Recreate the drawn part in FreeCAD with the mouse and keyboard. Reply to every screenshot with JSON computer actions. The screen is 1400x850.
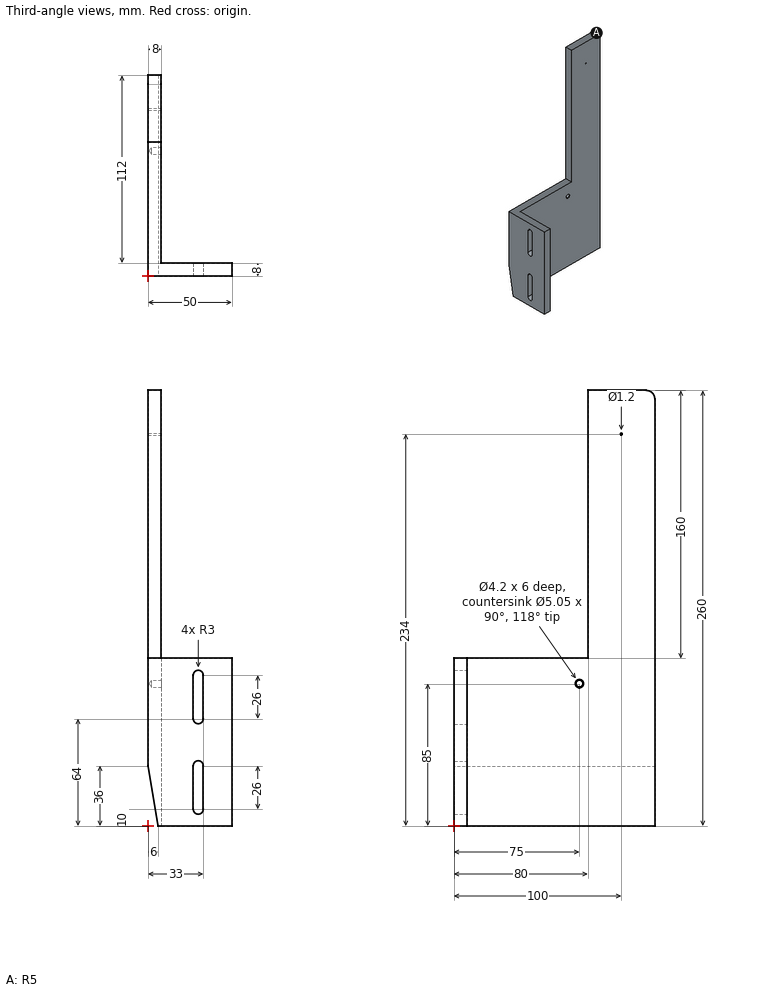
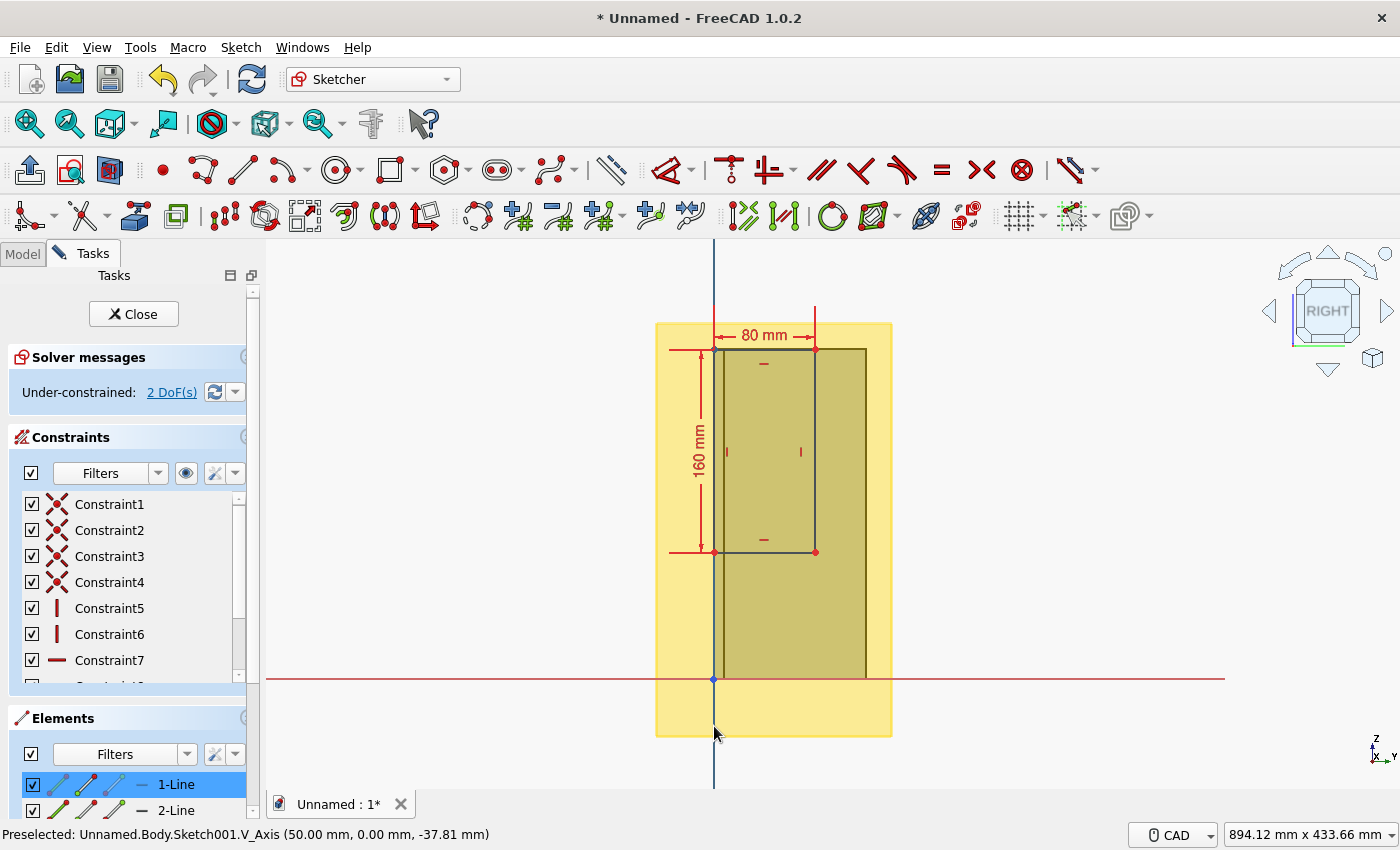
{"action": "left_click", "coordinate": [730, 170]}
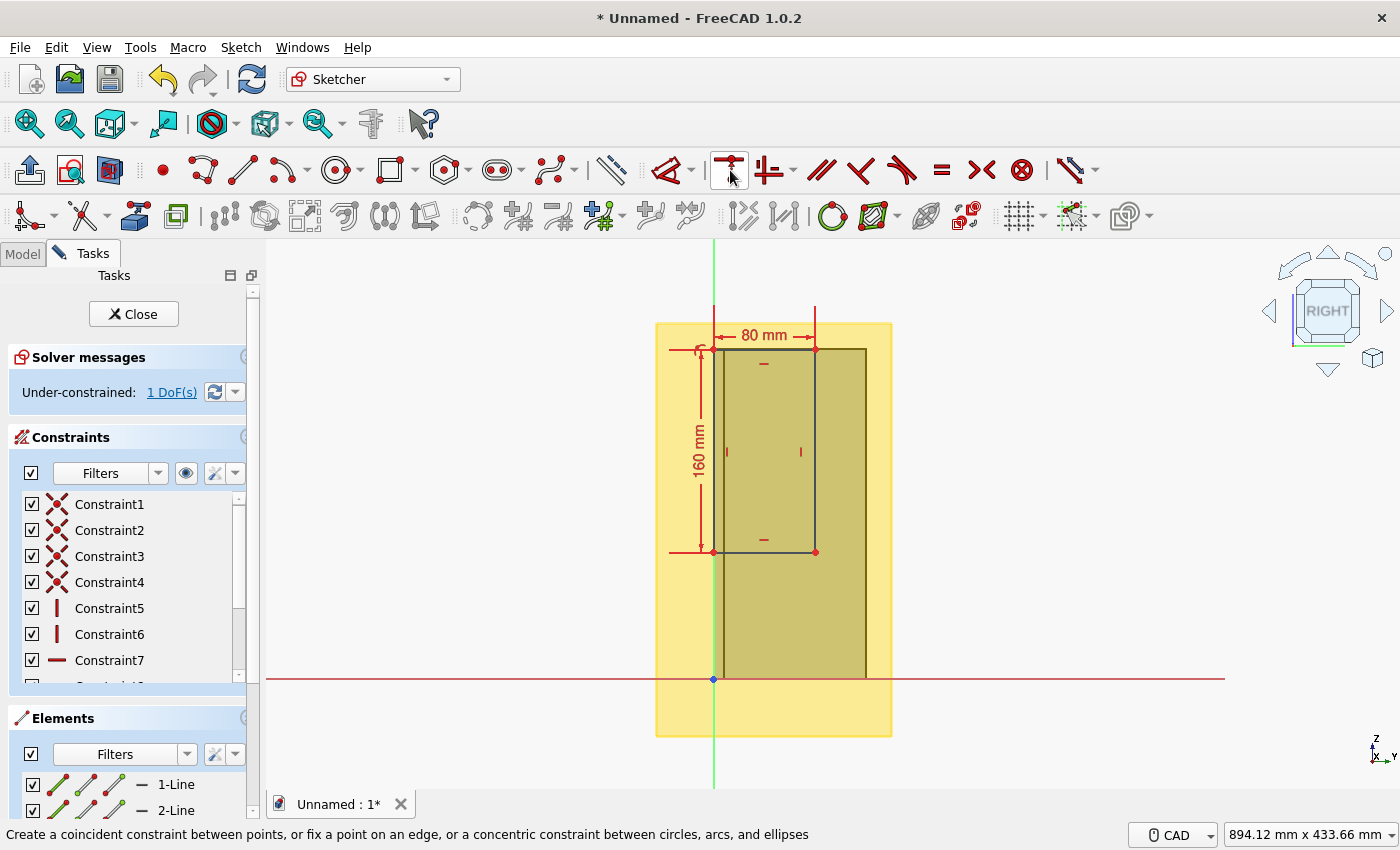
{"action": "left_click", "coordinate": [666, 170]}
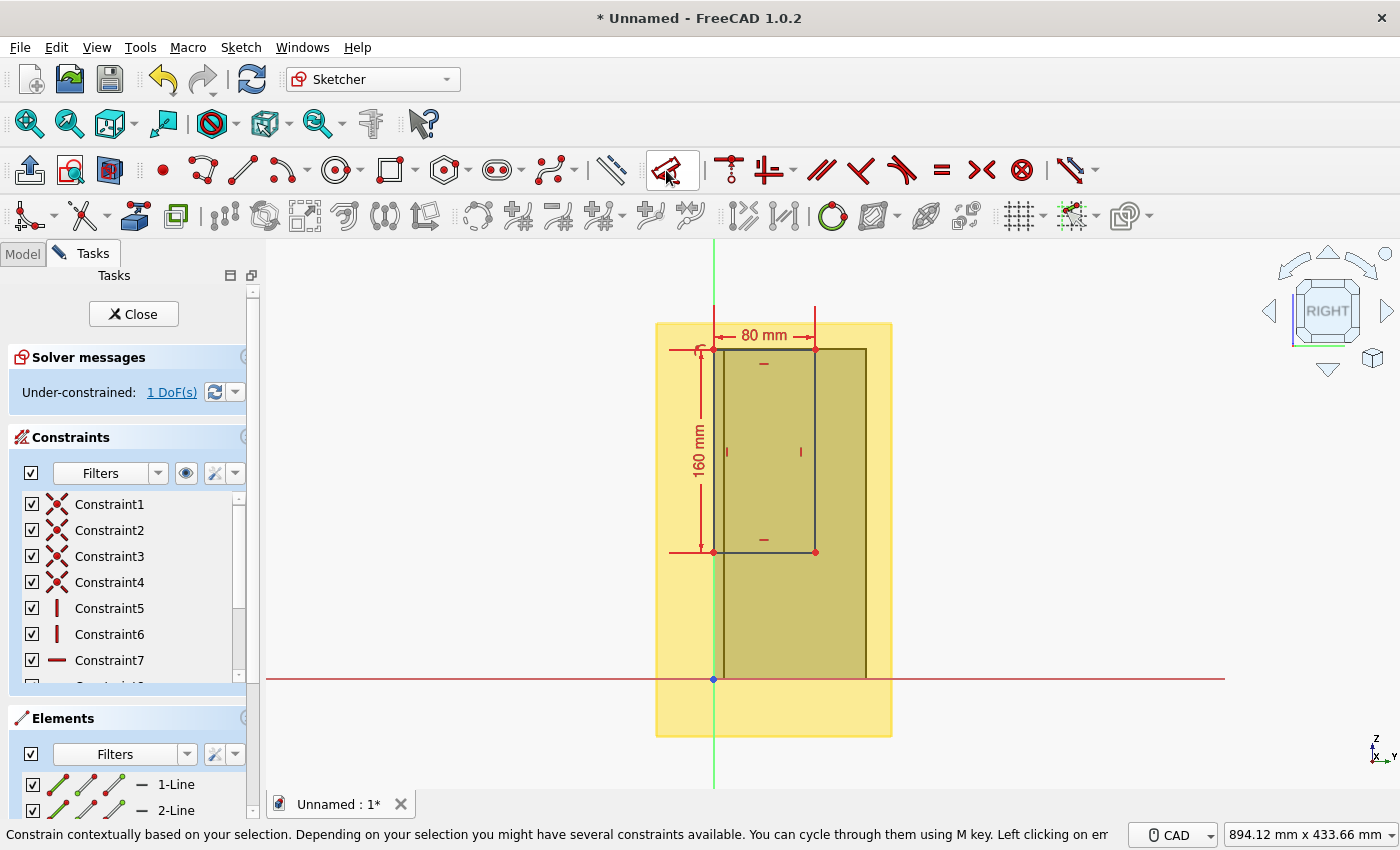
{"action": "left_click", "coordinate": [714, 350]}
{"action": "left_click", "coordinate": [680, 515]}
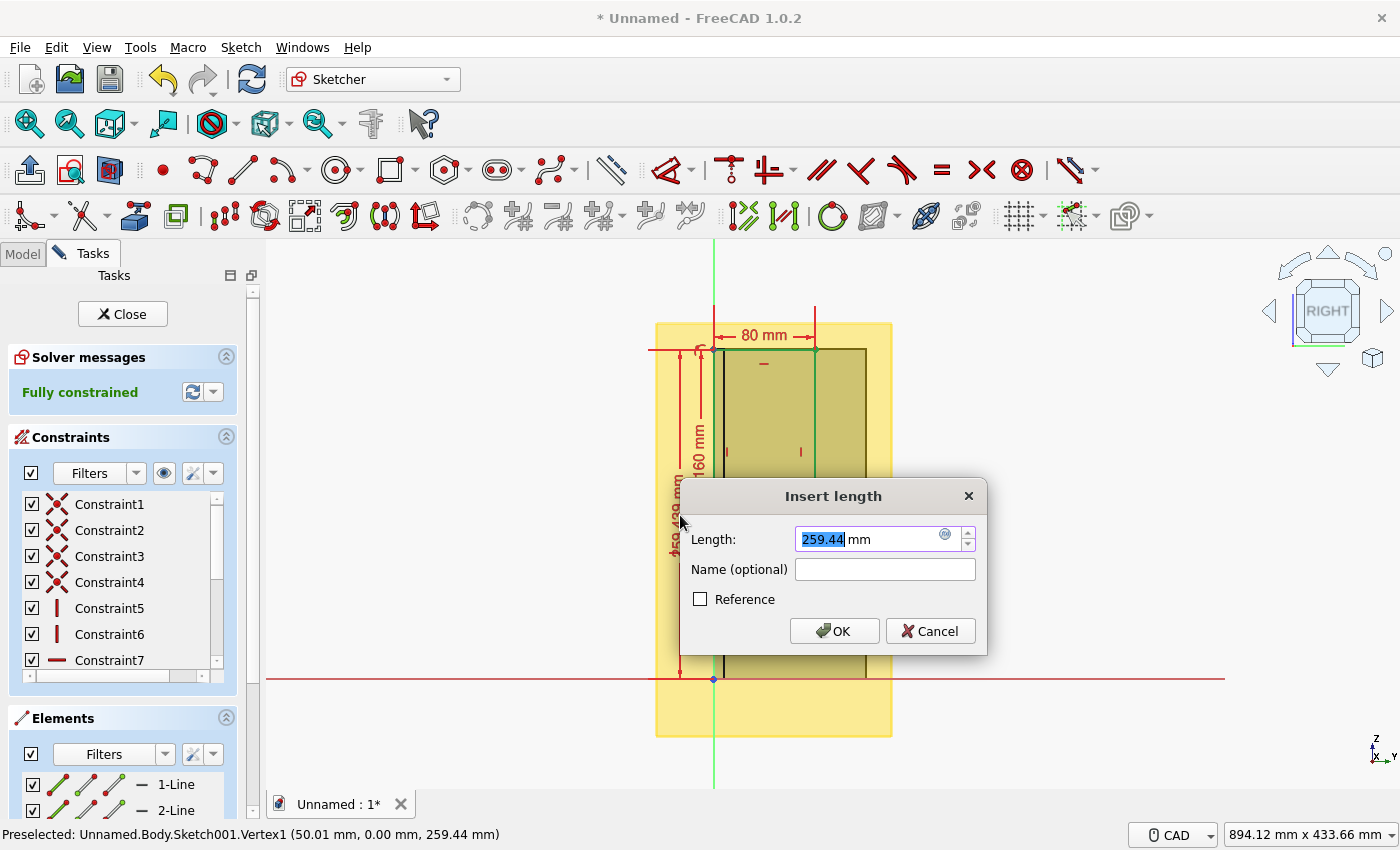
{"action": "type", "text": "260"}
{"action": "key", "text": "Return"}
{"action": "key", "text": "Escape"}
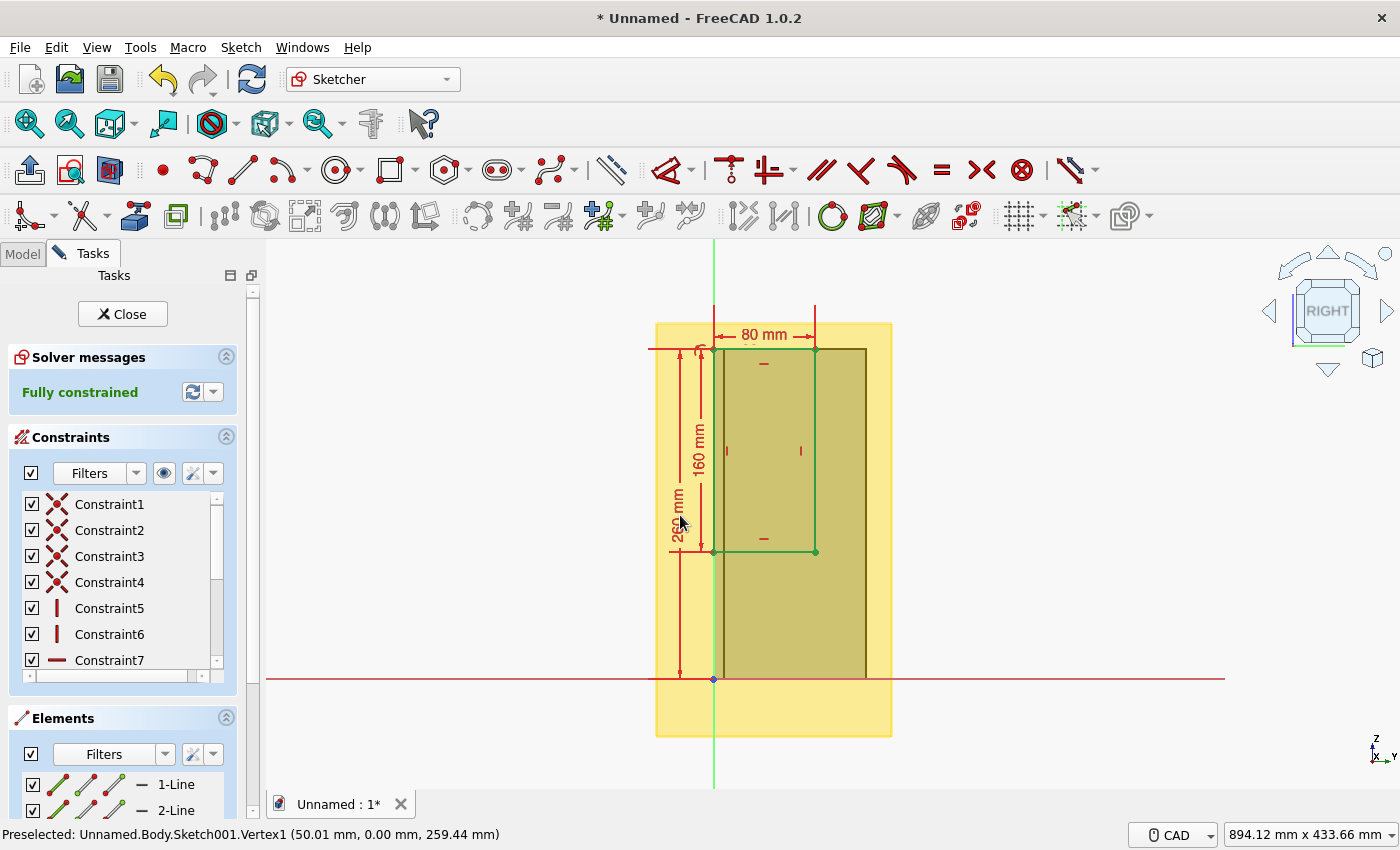
{"action": "left_click", "coordinate": [123, 314]}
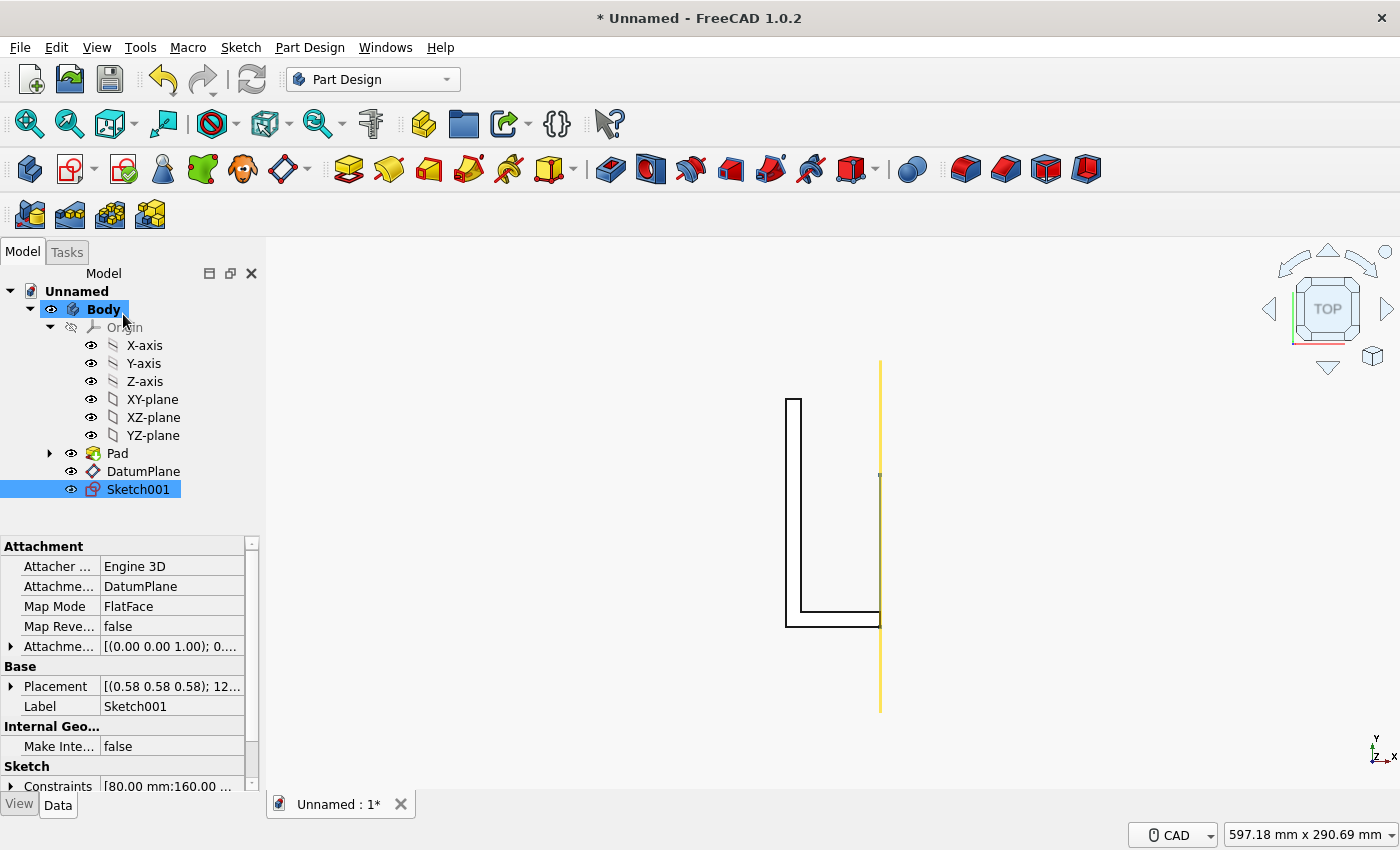
{"action": "left_click", "coordinate": [612, 170]}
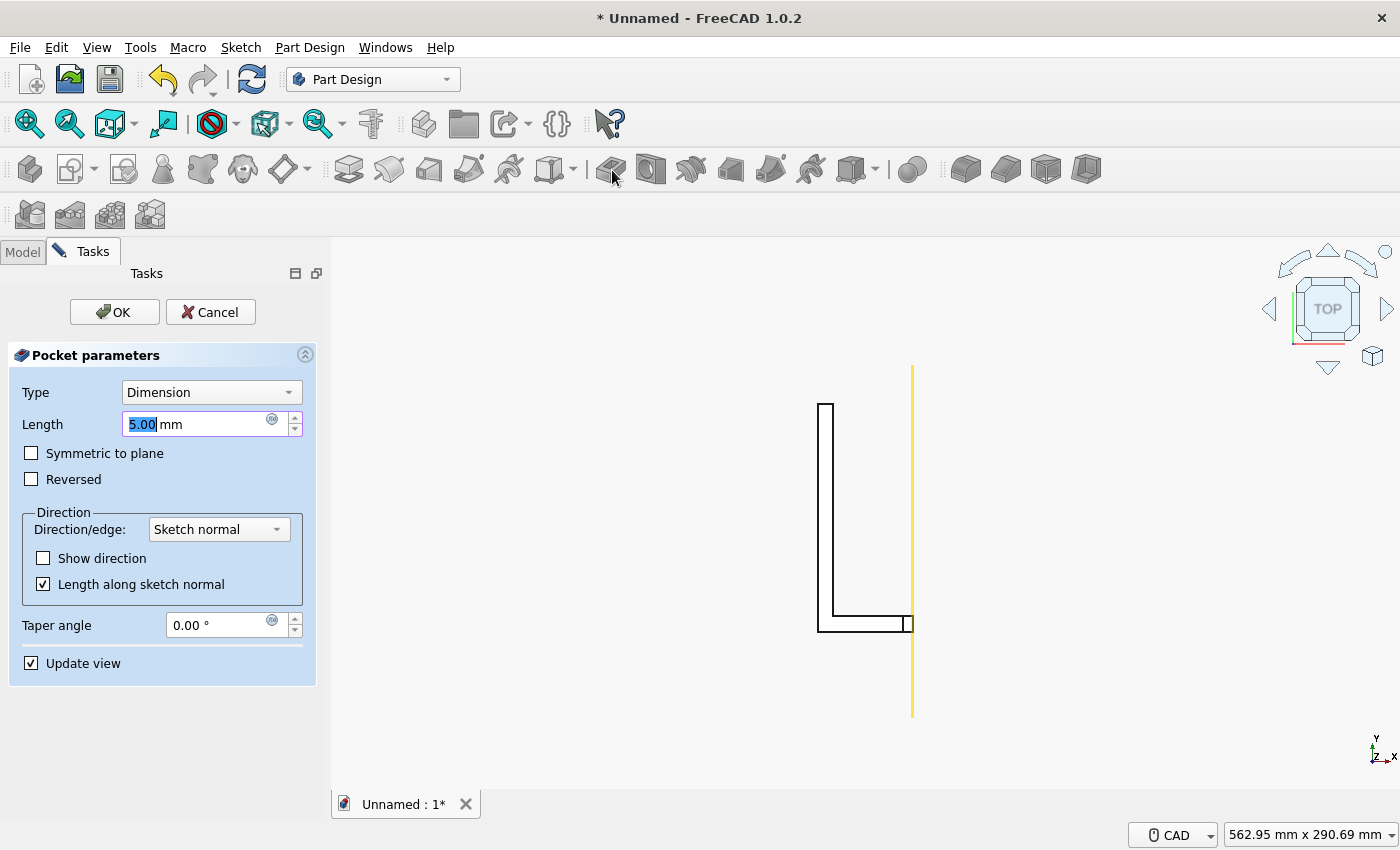
{"action": "left_click", "coordinate": [212, 392]}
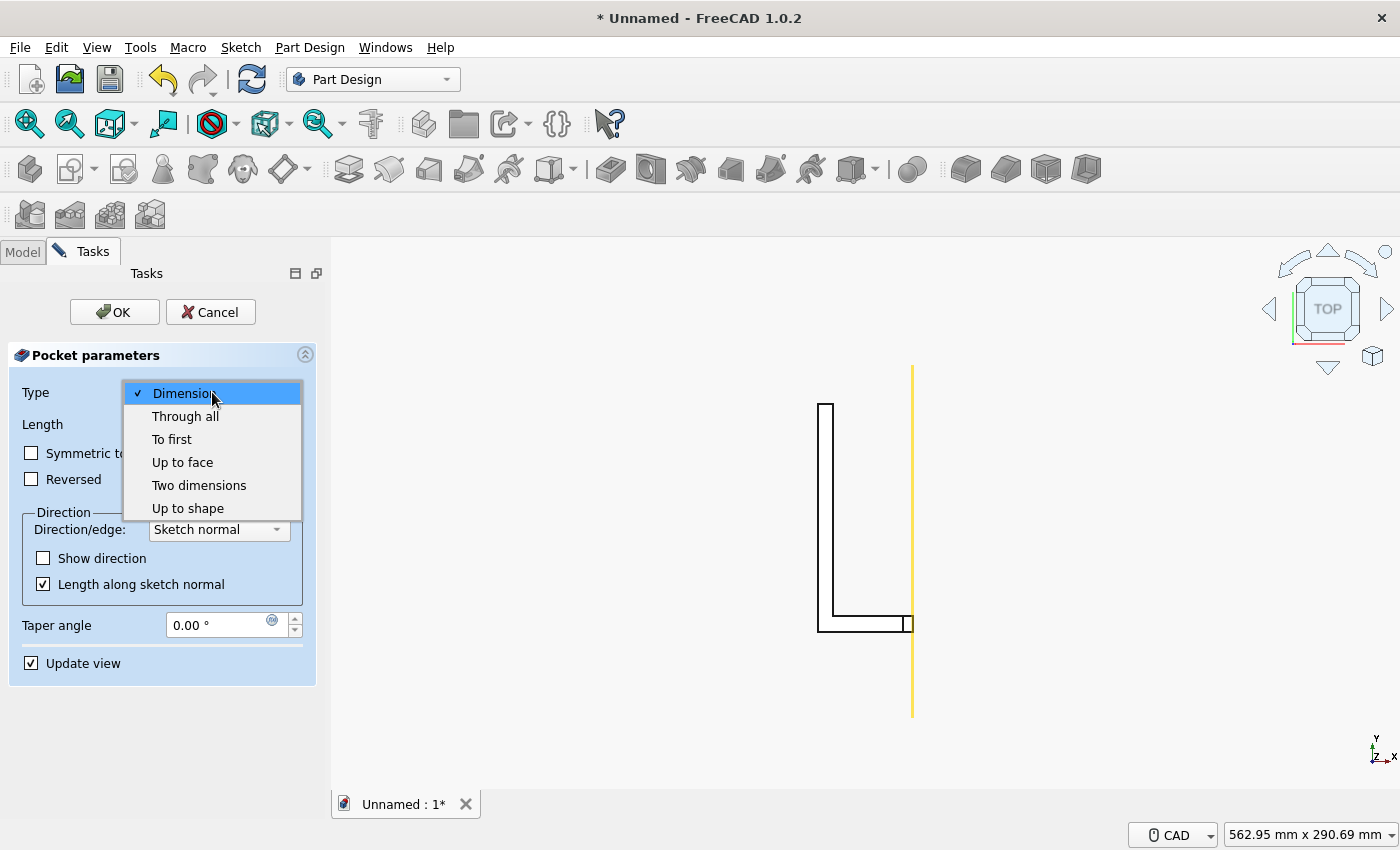
{"action": "left_click", "coordinate": [212, 416]}